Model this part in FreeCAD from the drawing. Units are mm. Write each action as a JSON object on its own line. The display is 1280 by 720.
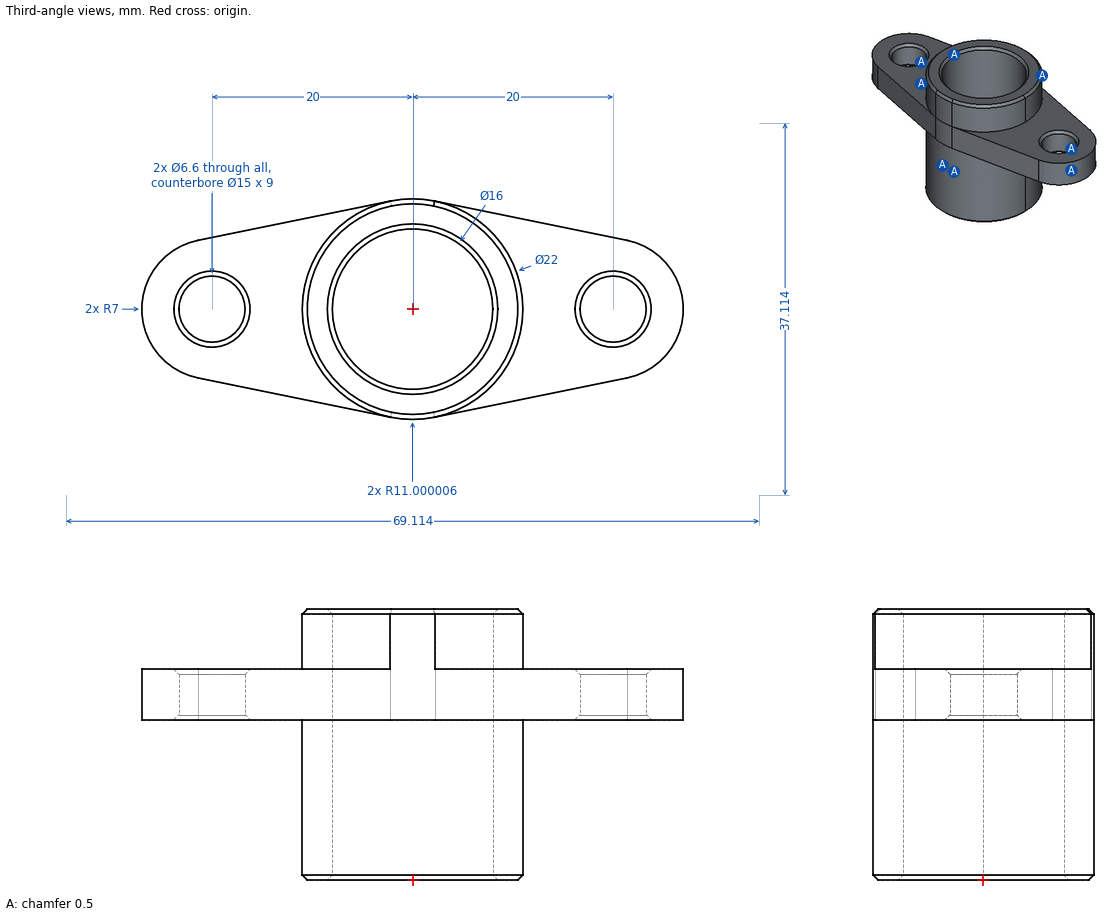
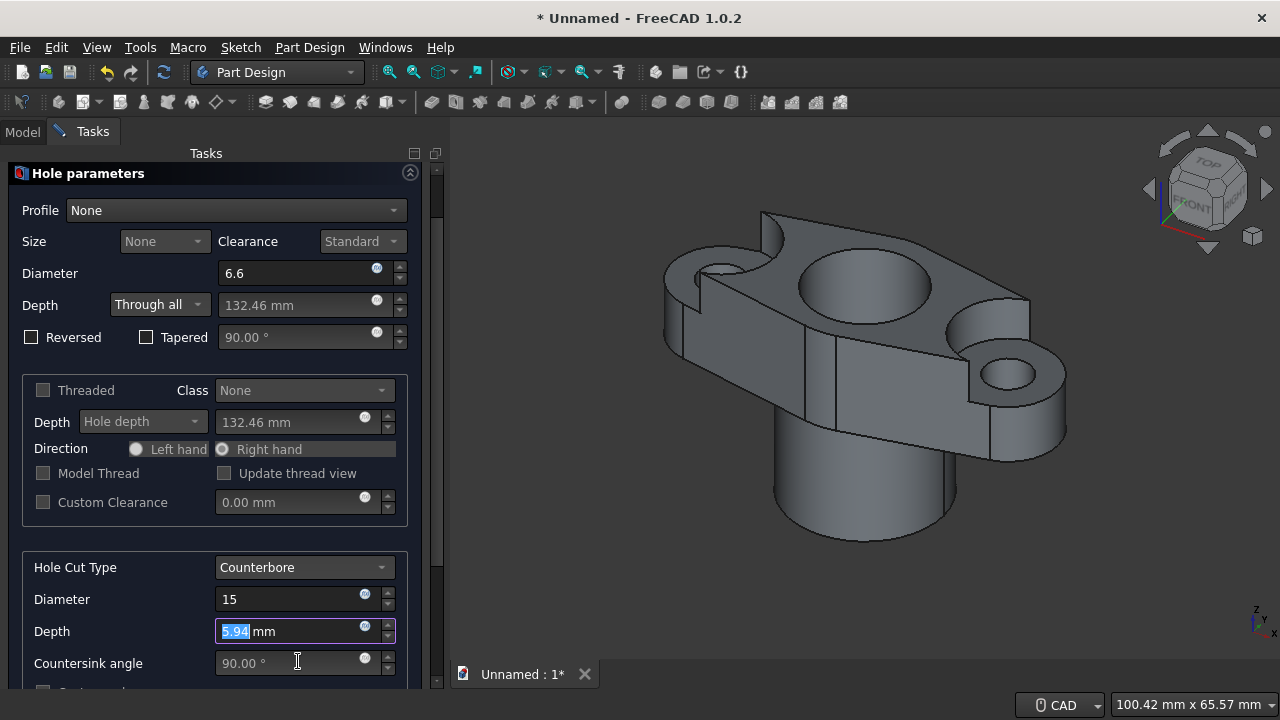
{"action": "type", "text": "9"}
{"action": "key", "text": "Tab"}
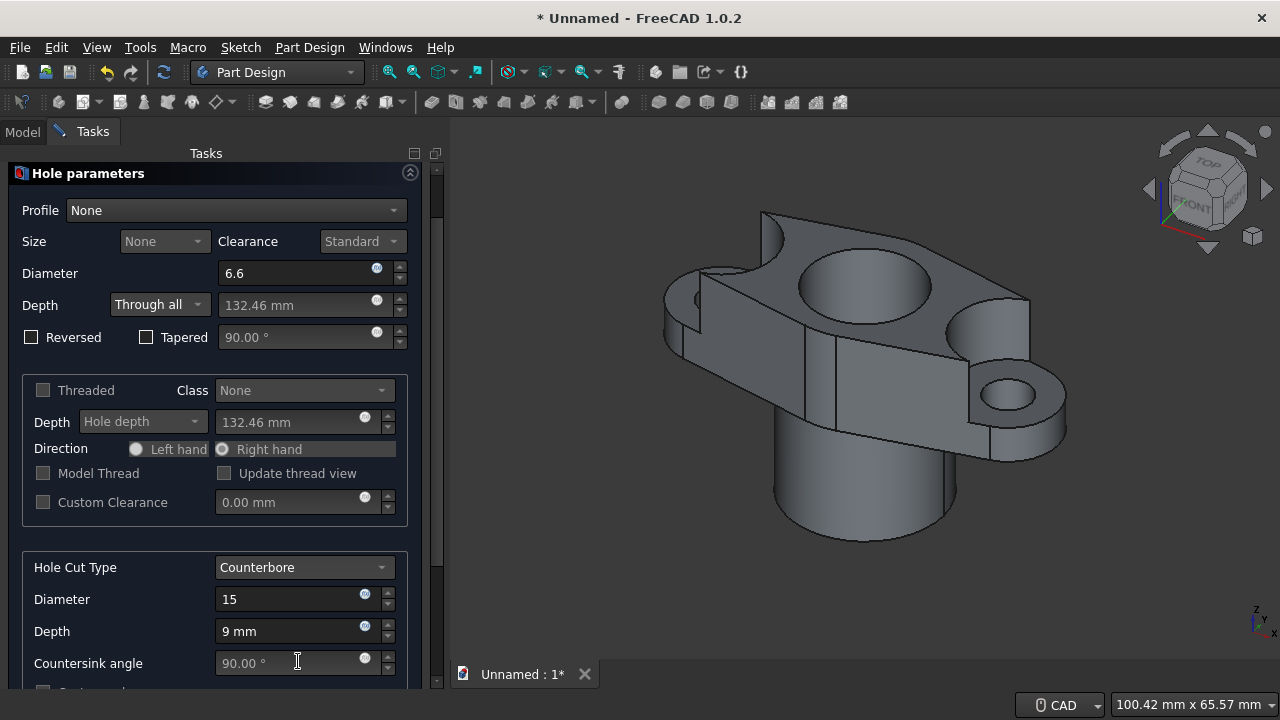
{"action": "scroll", "coordinate": [437, 426], "scroll_direction": "up", "scroll_amount": 2}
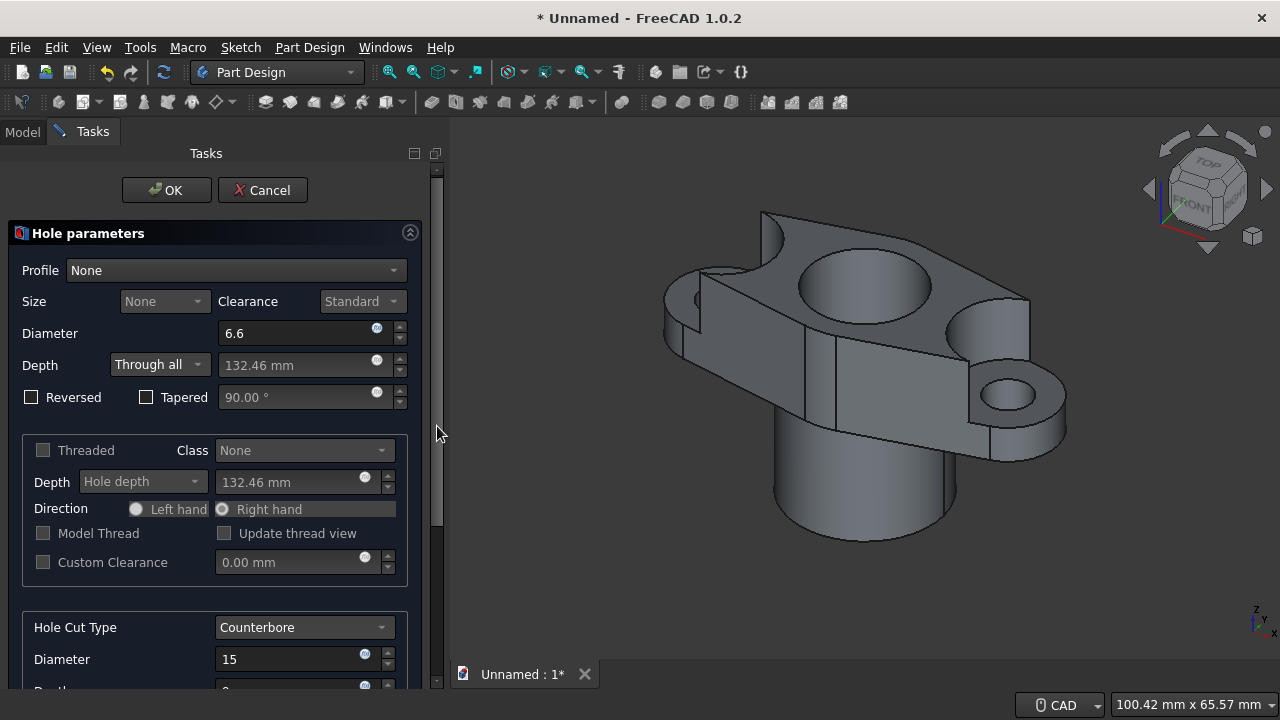
{"action": "left_click", "coordinate": [167, 192]}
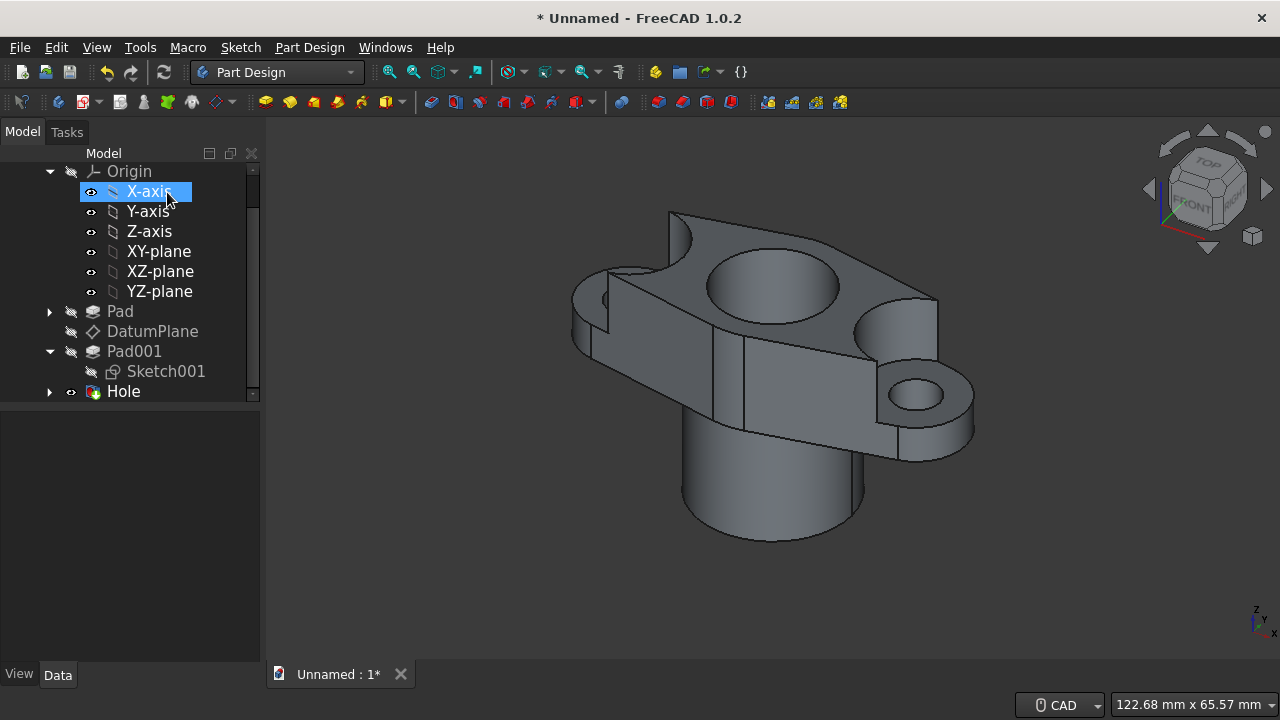
{"action": "left_click", "coordinate": [824, 337]}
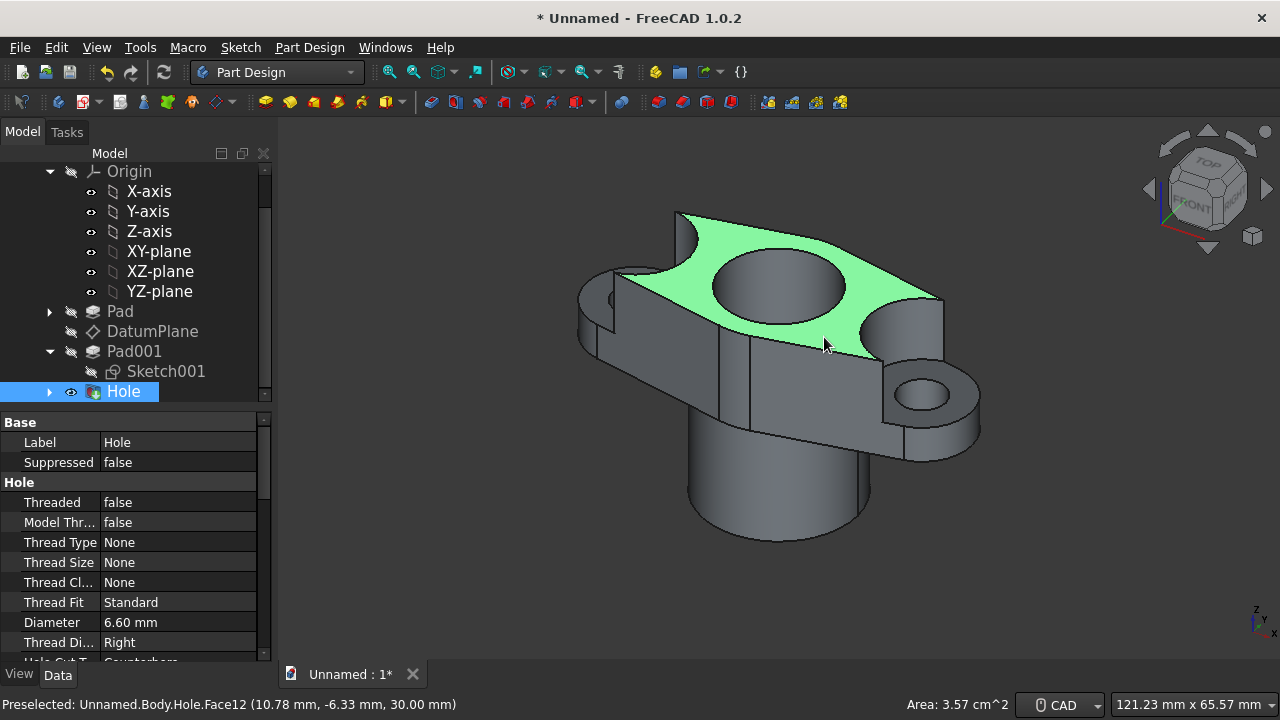
{"action": "left_click", "coordinate": [84, 102]}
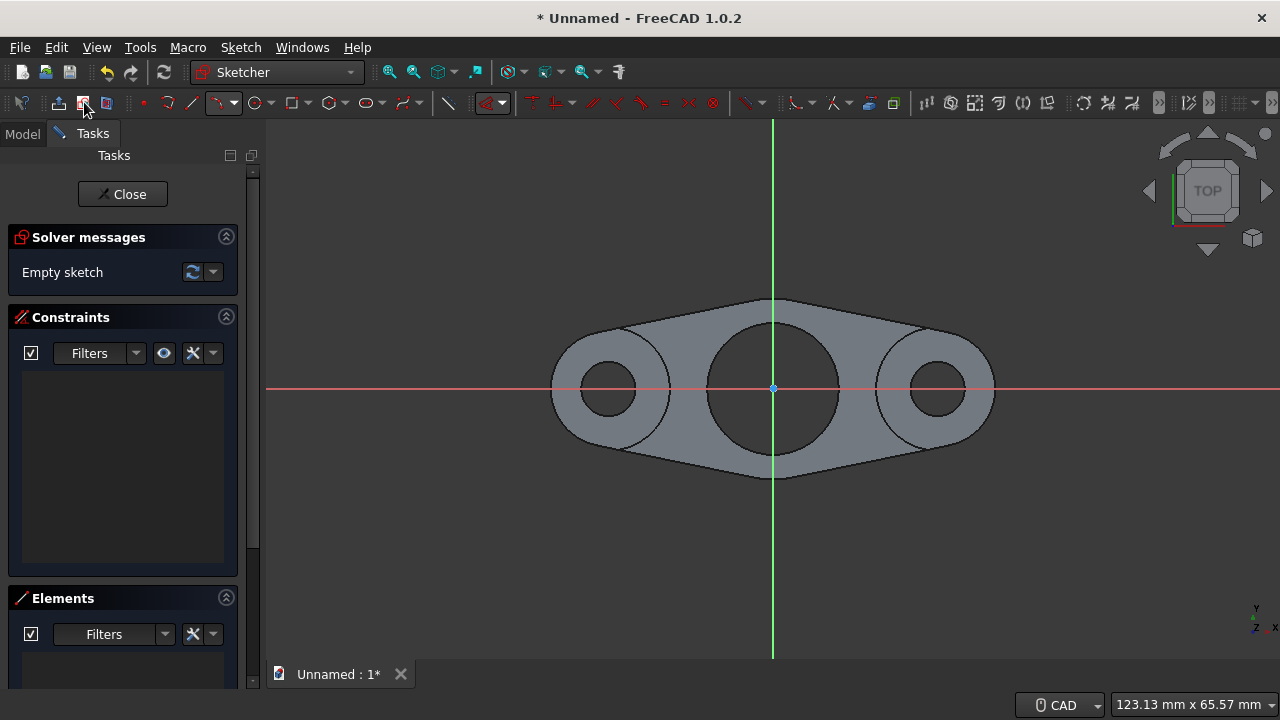
{"action": "key", "text": "g v"}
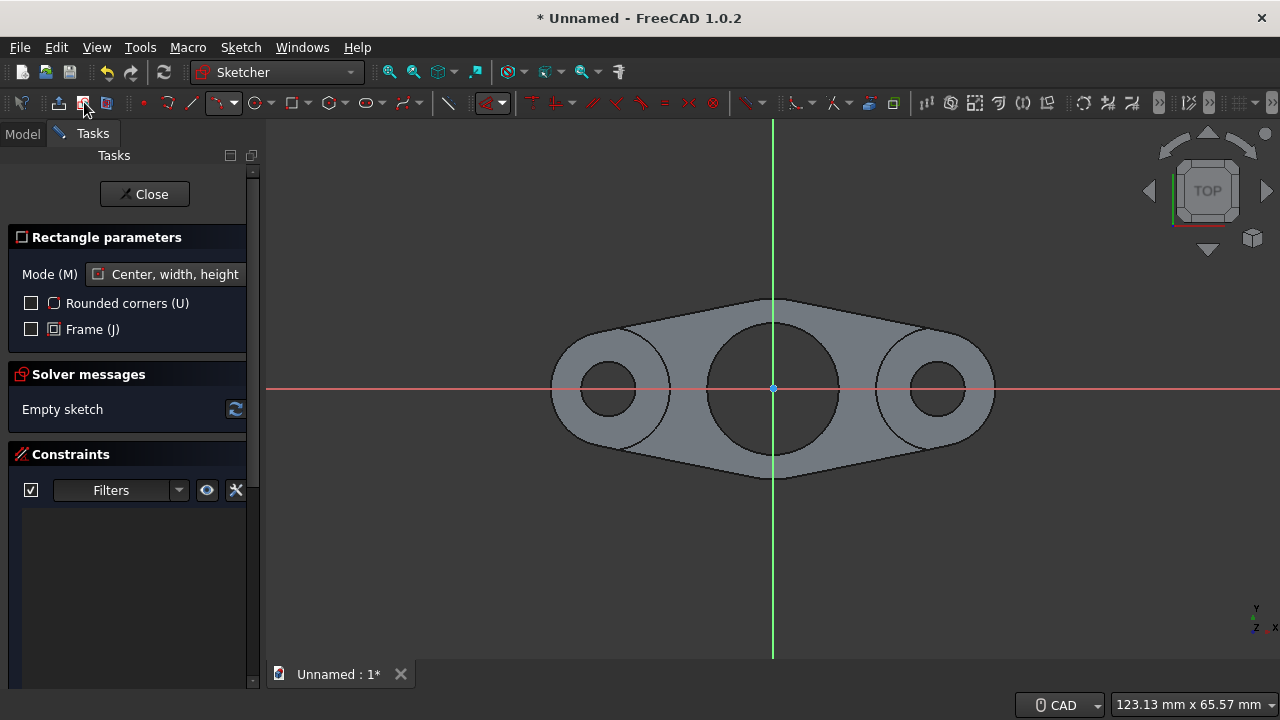
{"action": "left_click", "coordinate": [773, 389]}
{"action": "left_click", "coordinate": [1058, 236]}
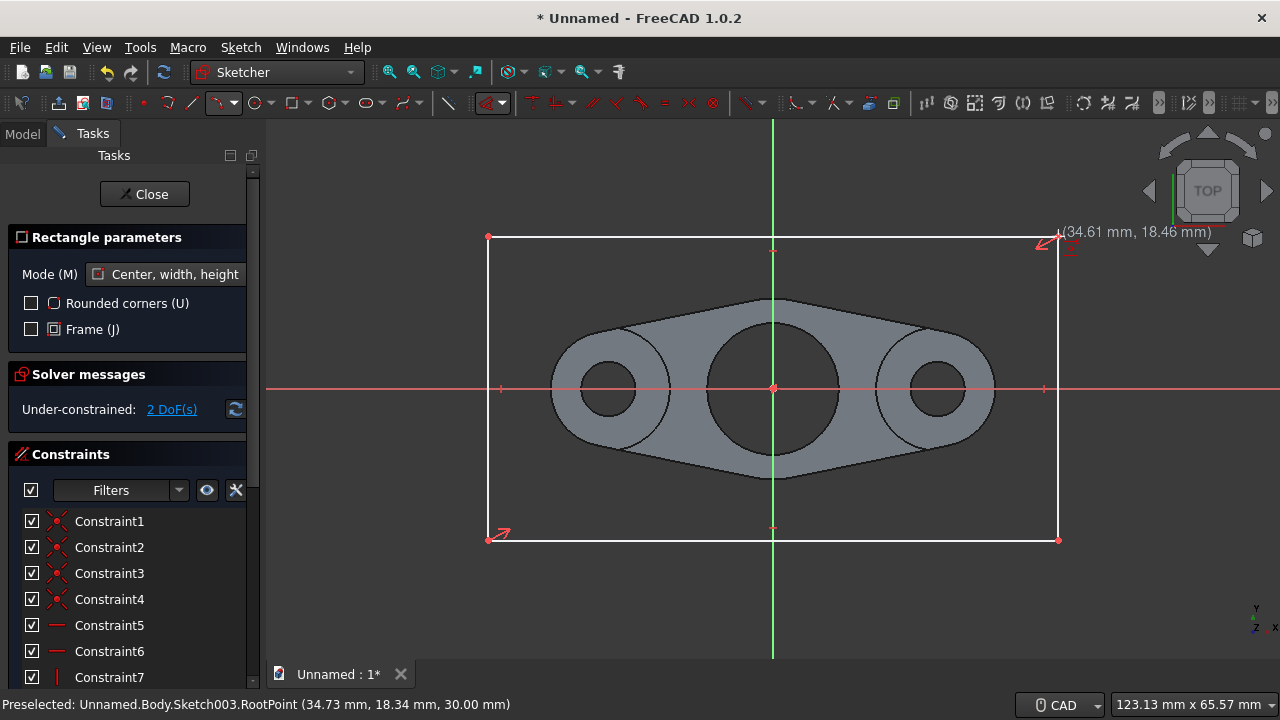
{"action": "left_click", "coordinate": [256, 104]}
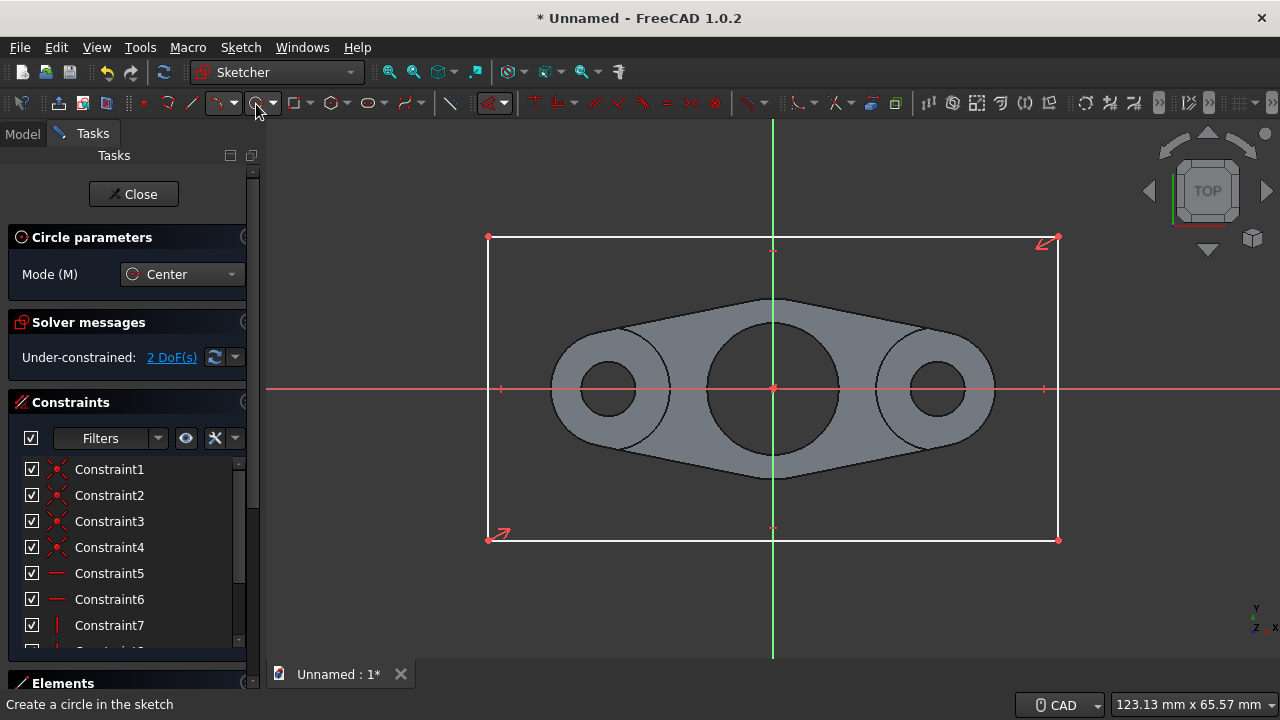
{"action": "left_click", "coordinate": [773, 389]}
{"action": "left_click", "coordinate": [837, 325]}
{"action": "key", "text": "Escape"}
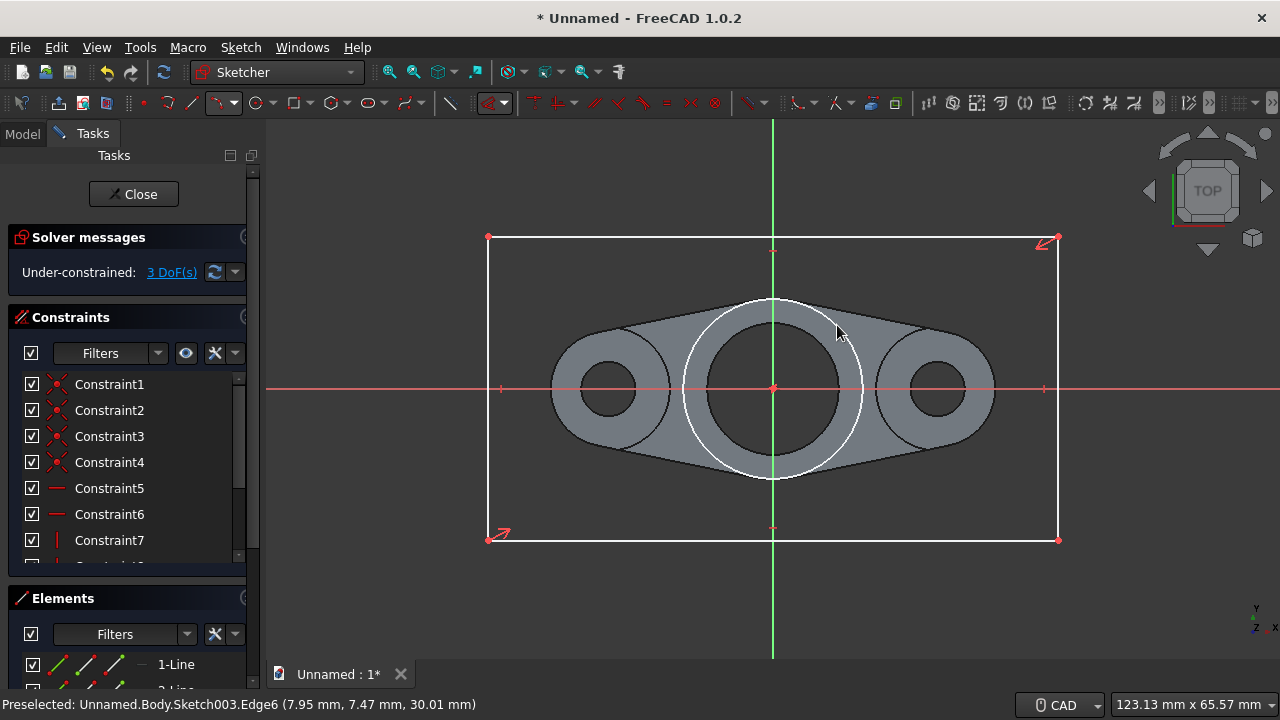
{"action": "left_click", "coordinate": [836, 325]}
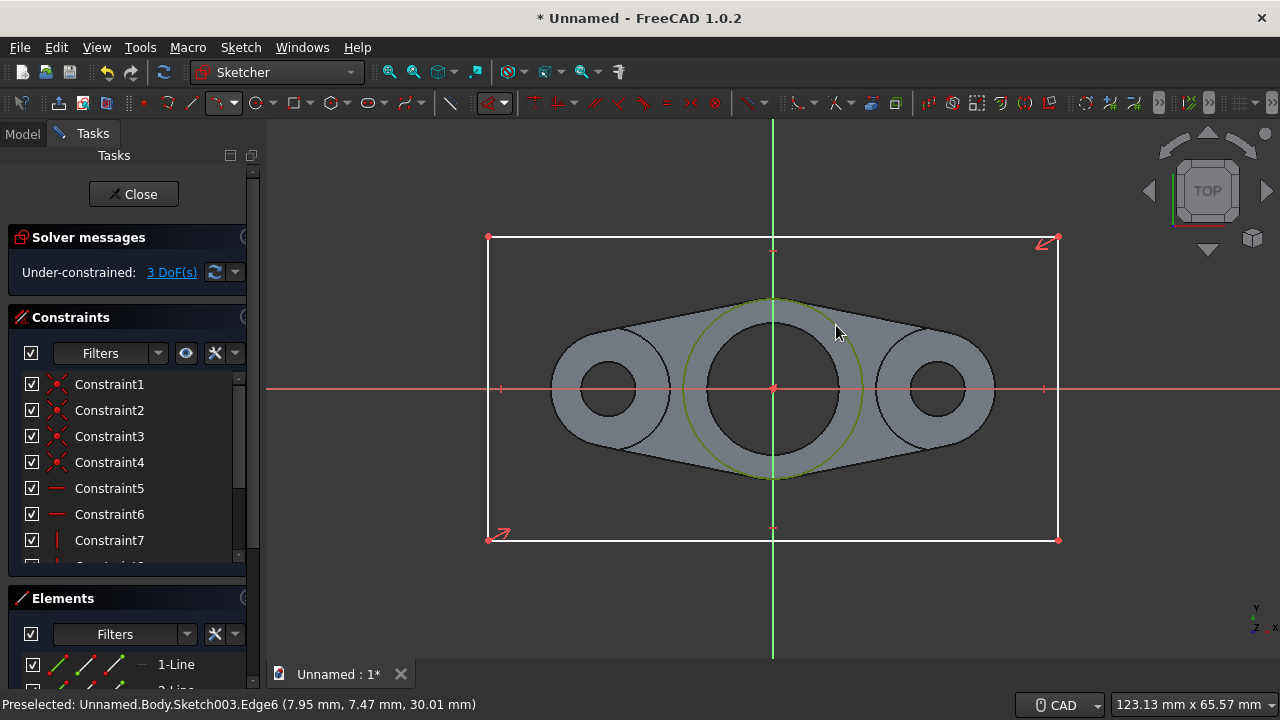
{"action": "key", "text": "k o"}